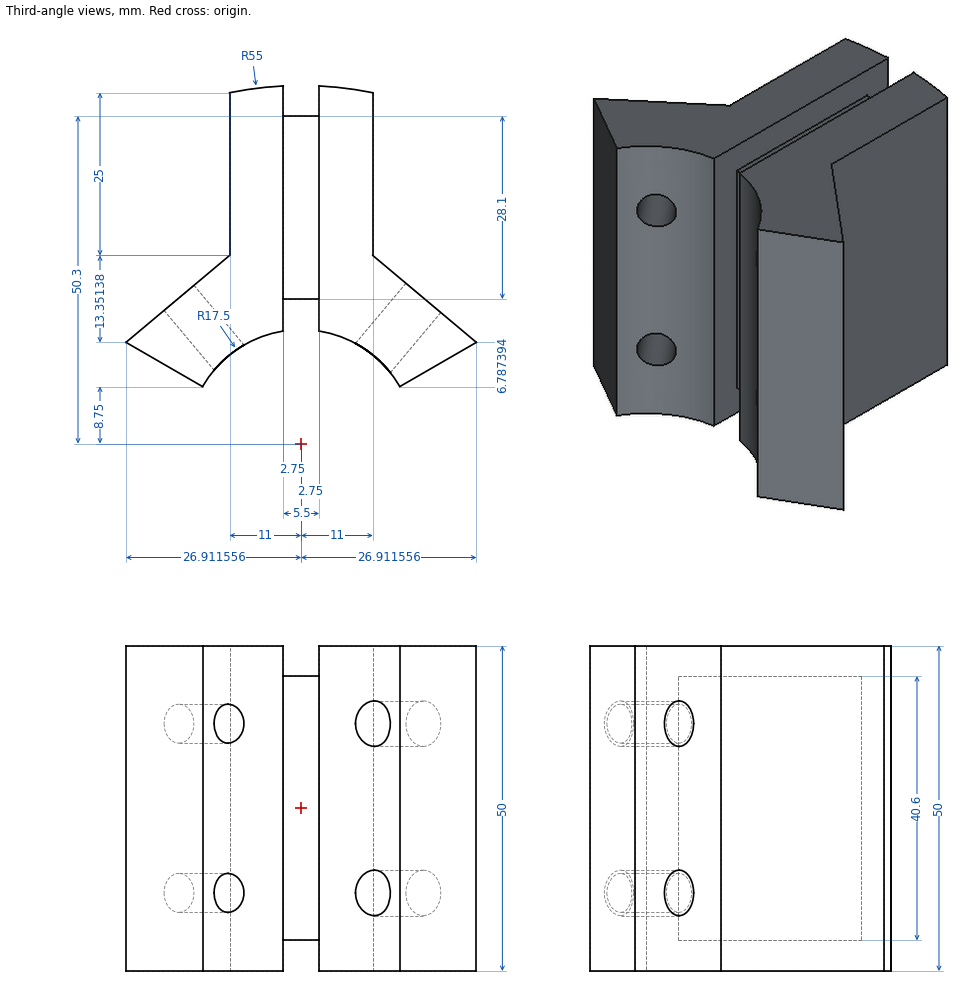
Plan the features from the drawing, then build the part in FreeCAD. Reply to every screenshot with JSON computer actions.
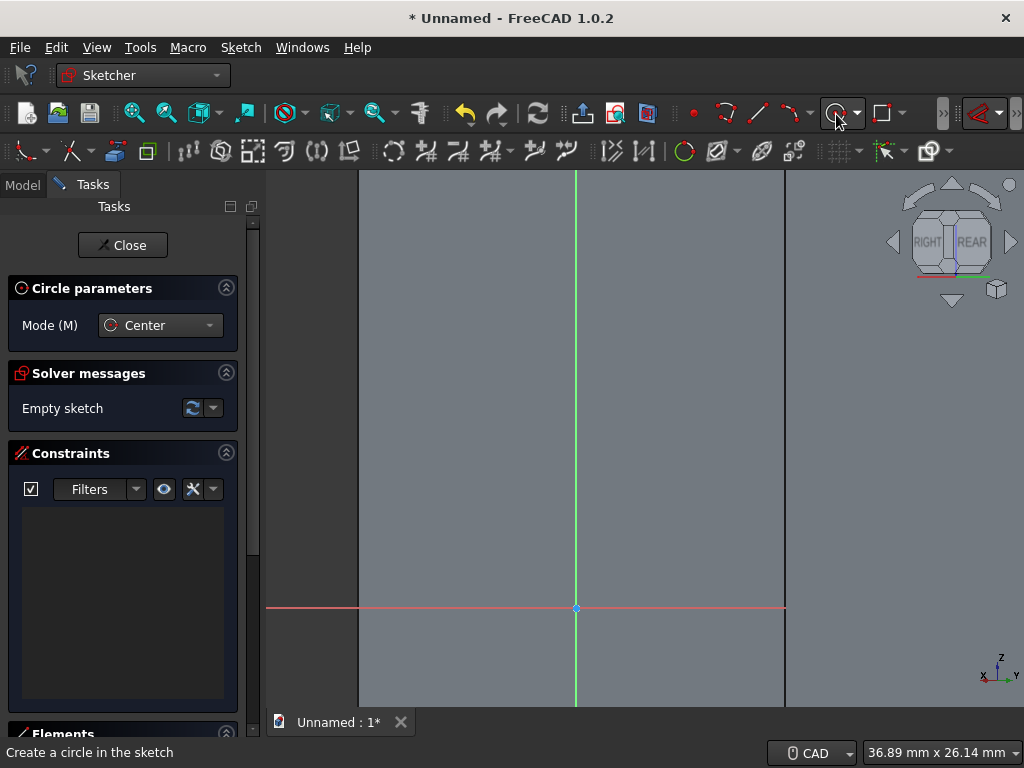
{"action": "left_click", "coordinate": [576, 341]}
{"action": "mouse_move", "coordinate": [627, 290]}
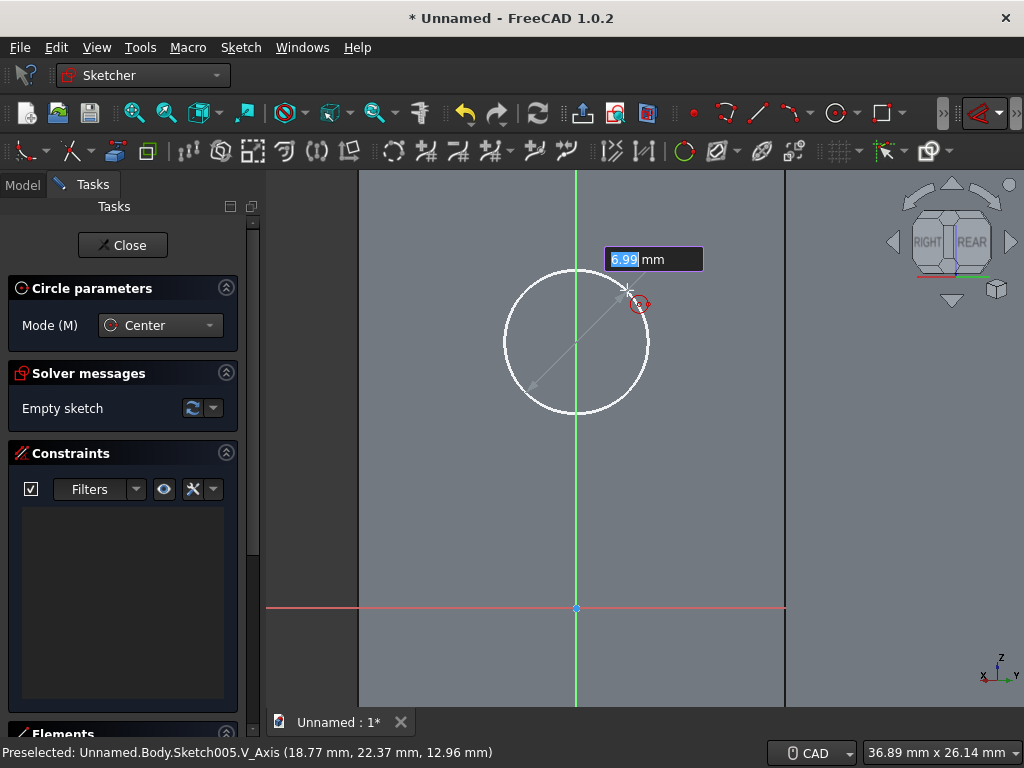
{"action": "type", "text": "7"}
{"action": "key", "text": "Return"}
{"action": "key", "text": "Escape"}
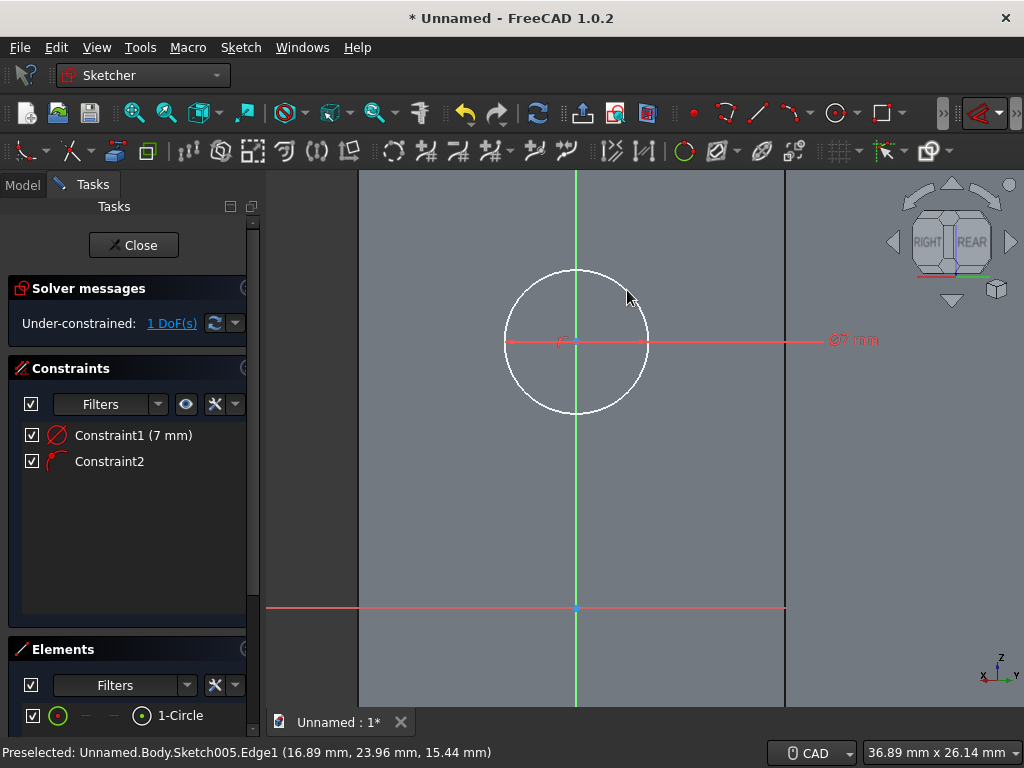
{"action": "left_click", "coordinate": [576, 342]}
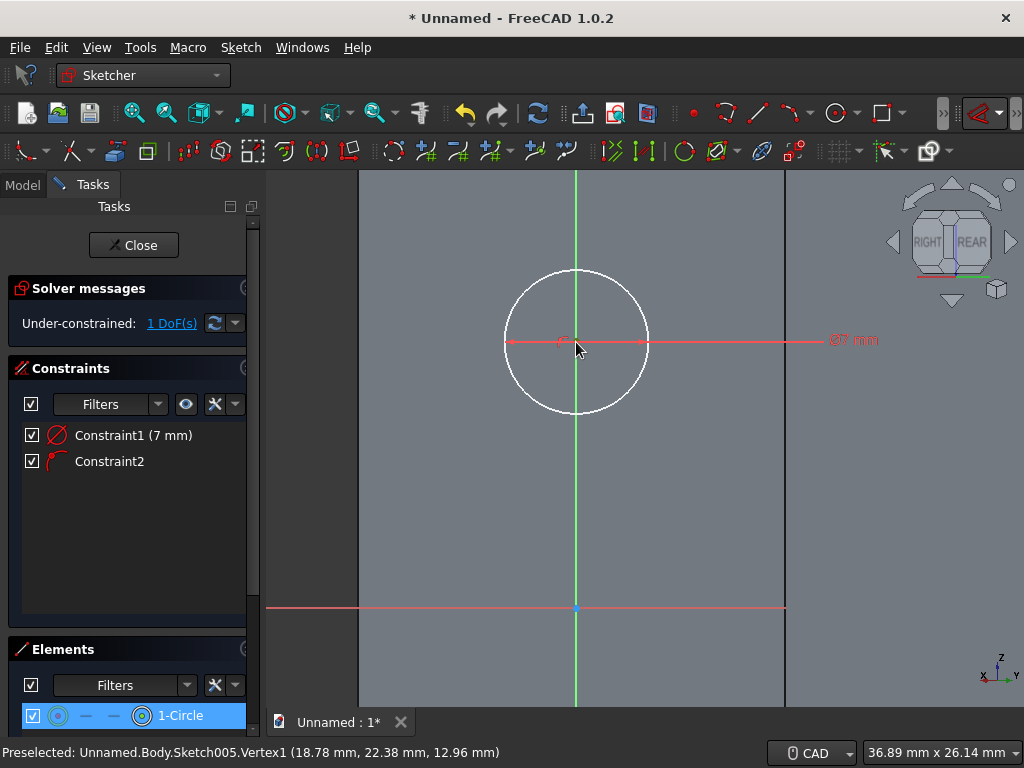
{"action": "left_click", "coordinate": [1002, 114]}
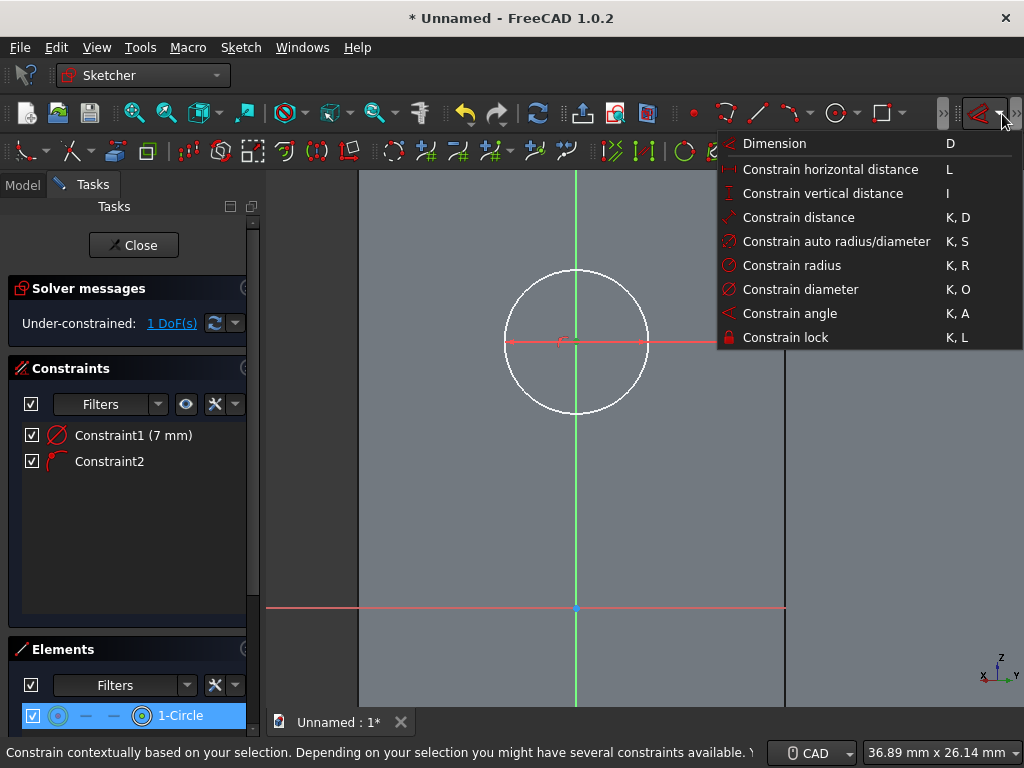
{"action": "left_click", "coordinate": [870, 193]}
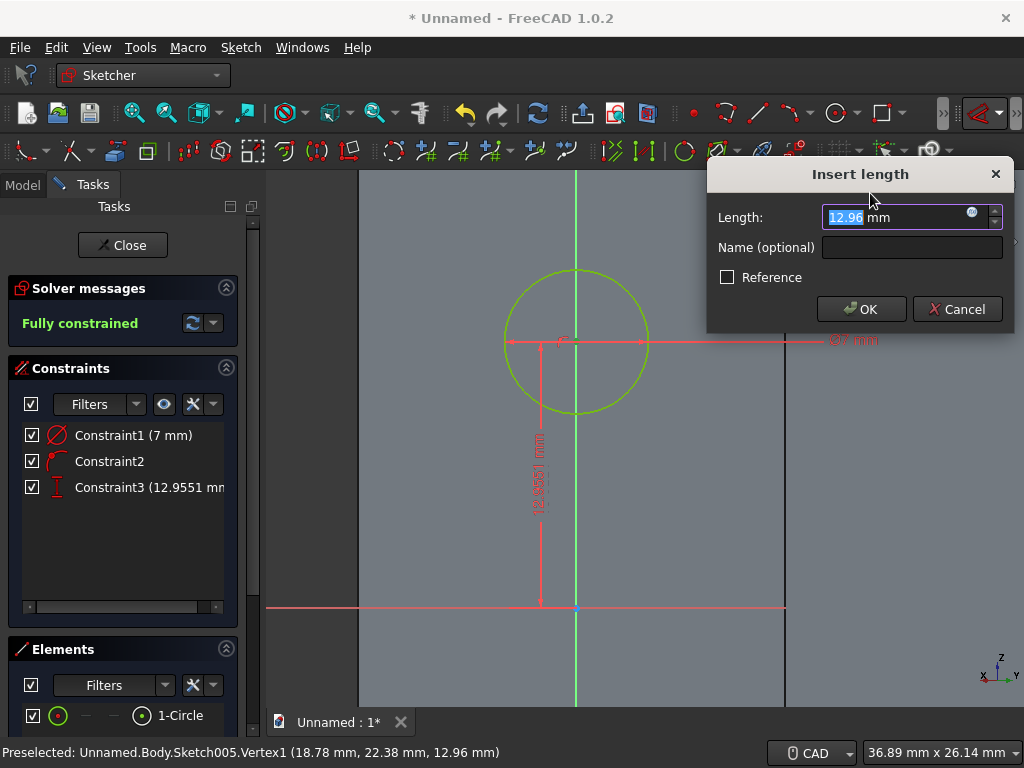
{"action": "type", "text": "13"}
{"action": "key", "text": "Return"}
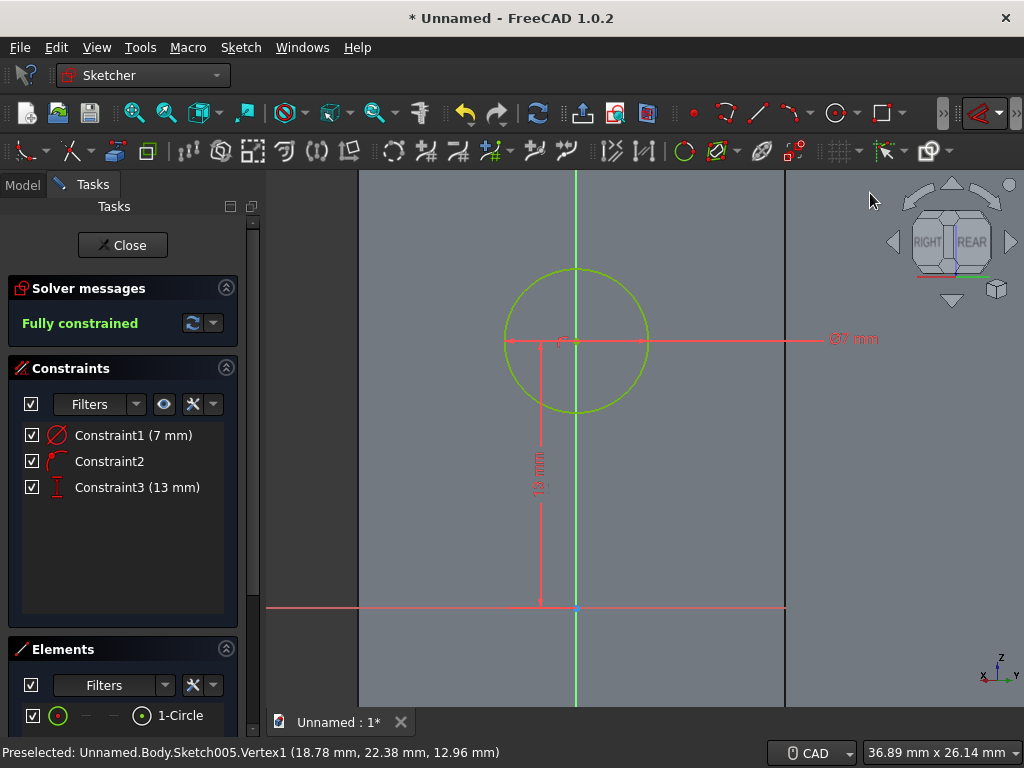
{"action": "left_click", "coordinate": [123, 245]}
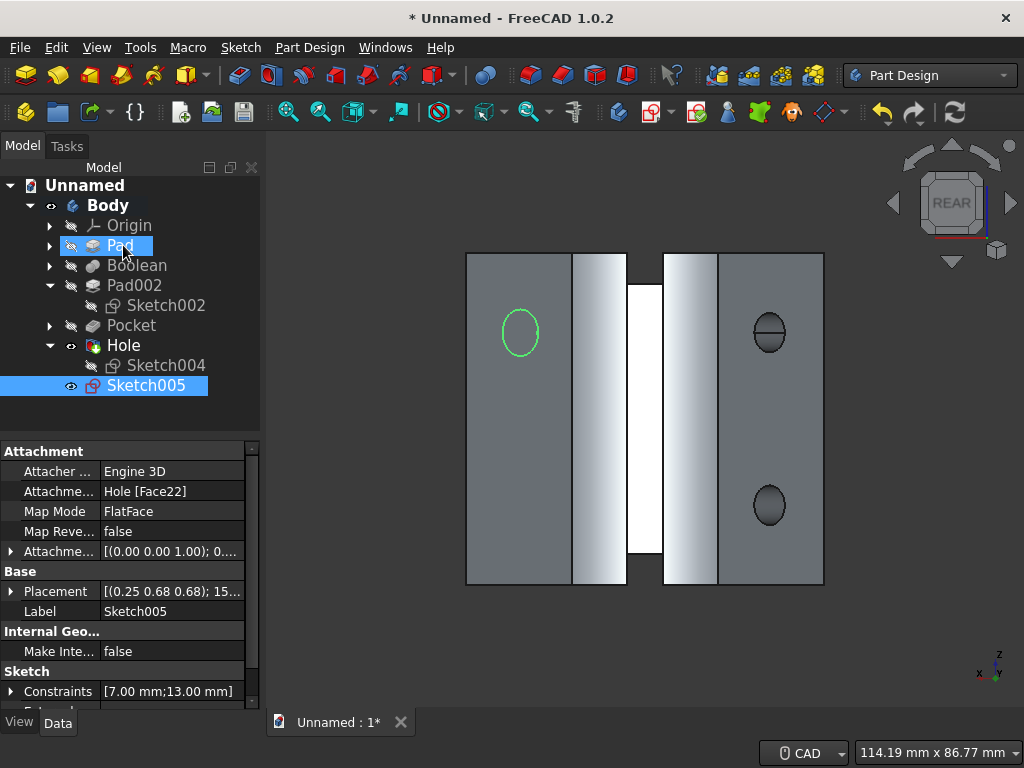
{"action": "left_click", "coordinate": [240, 76]}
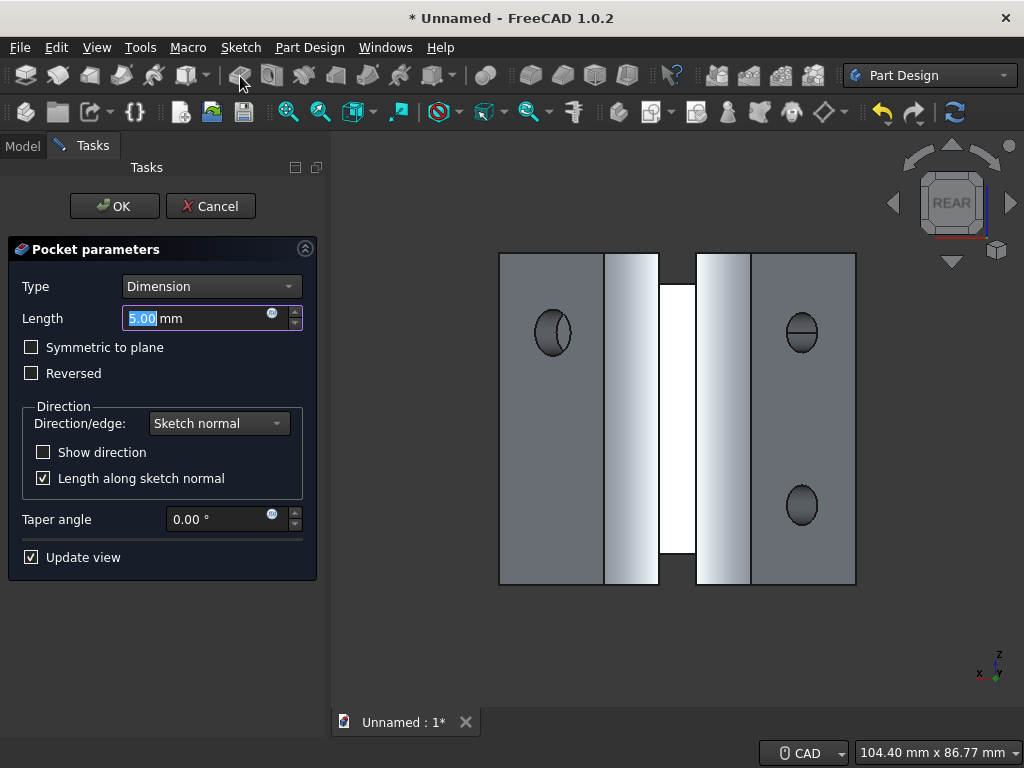
{"action": "left_click", "coordinate": [212, 286]}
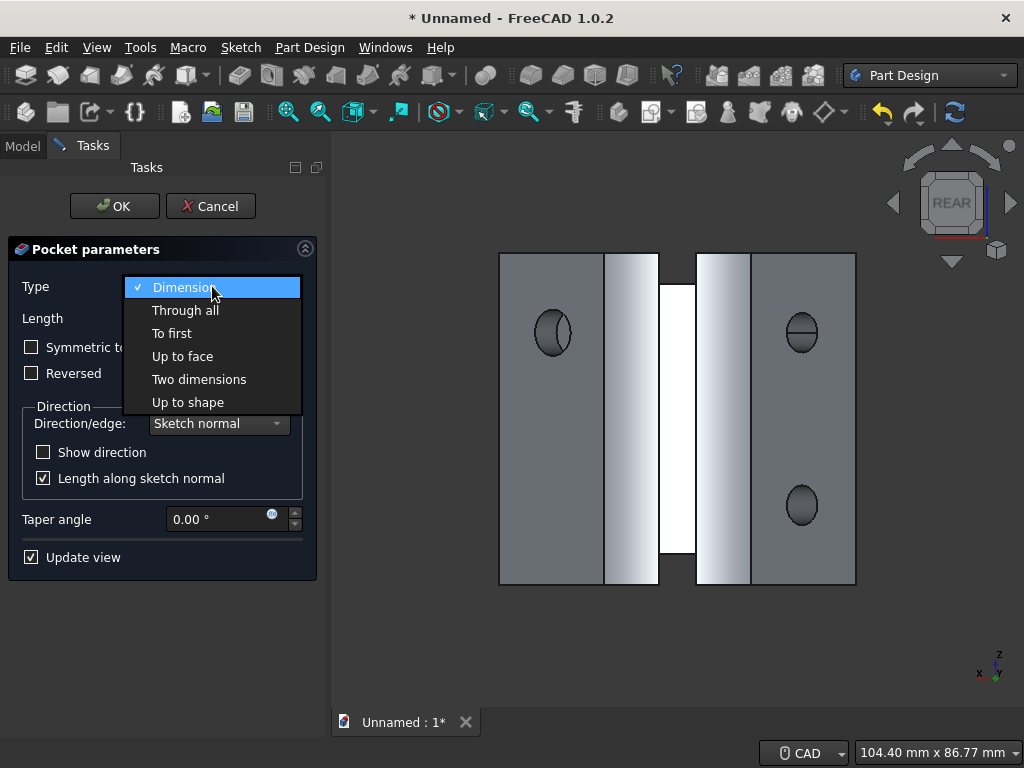
{"action": "left_click", "coordinate": [212, 310]}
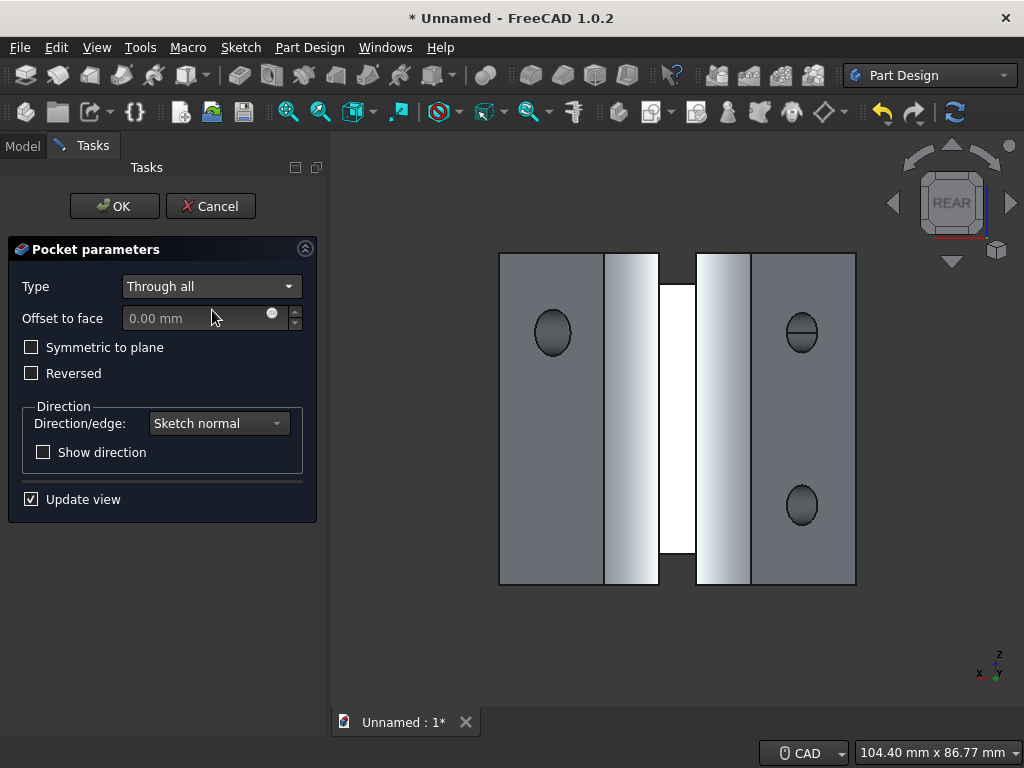
{"action": "left_click", "coordinate": [115, 206]}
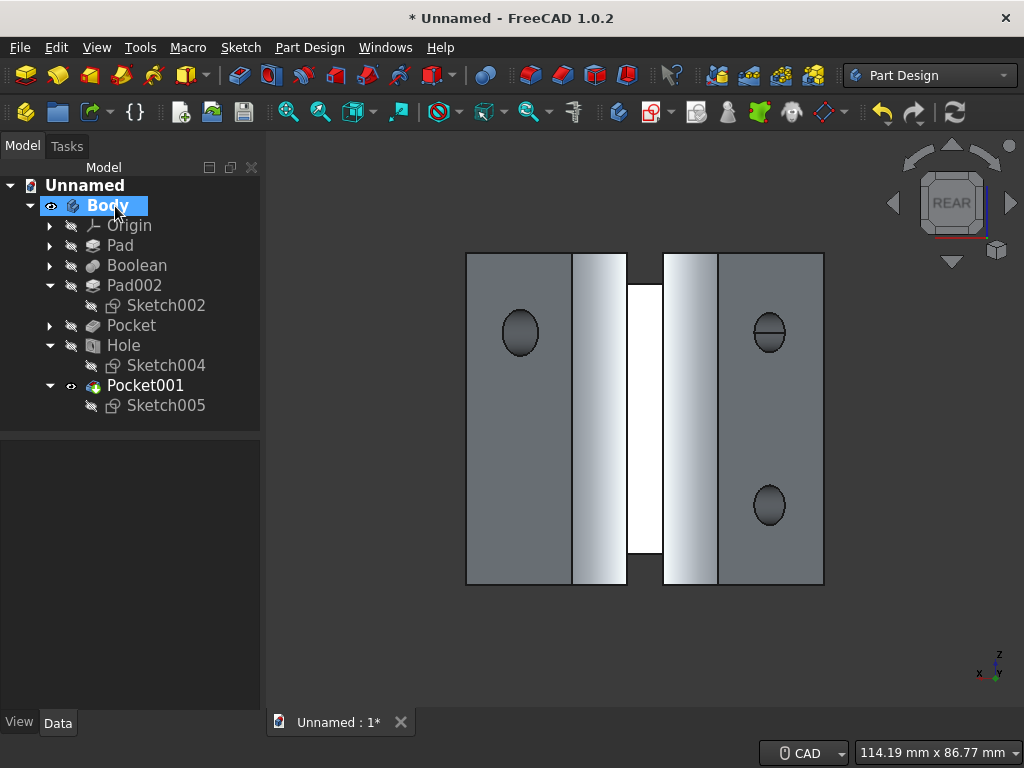
{"action": "left_click", "coordinate": [519, 465]}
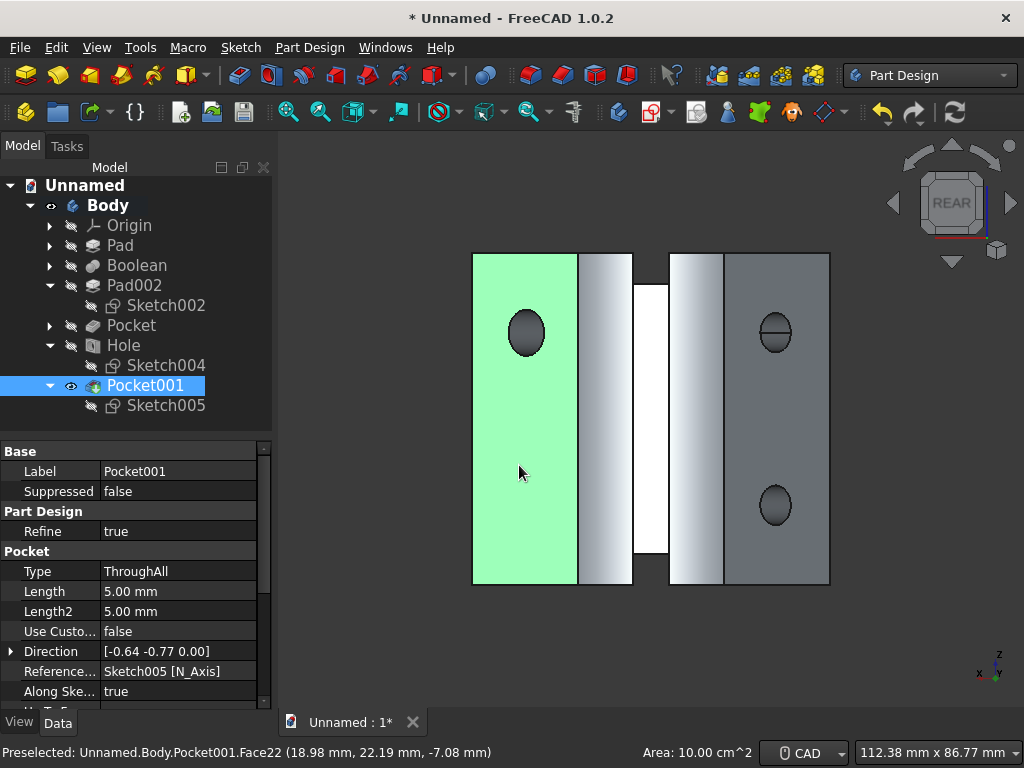
{"action": "left_click", "coordinate": [652, 112]}